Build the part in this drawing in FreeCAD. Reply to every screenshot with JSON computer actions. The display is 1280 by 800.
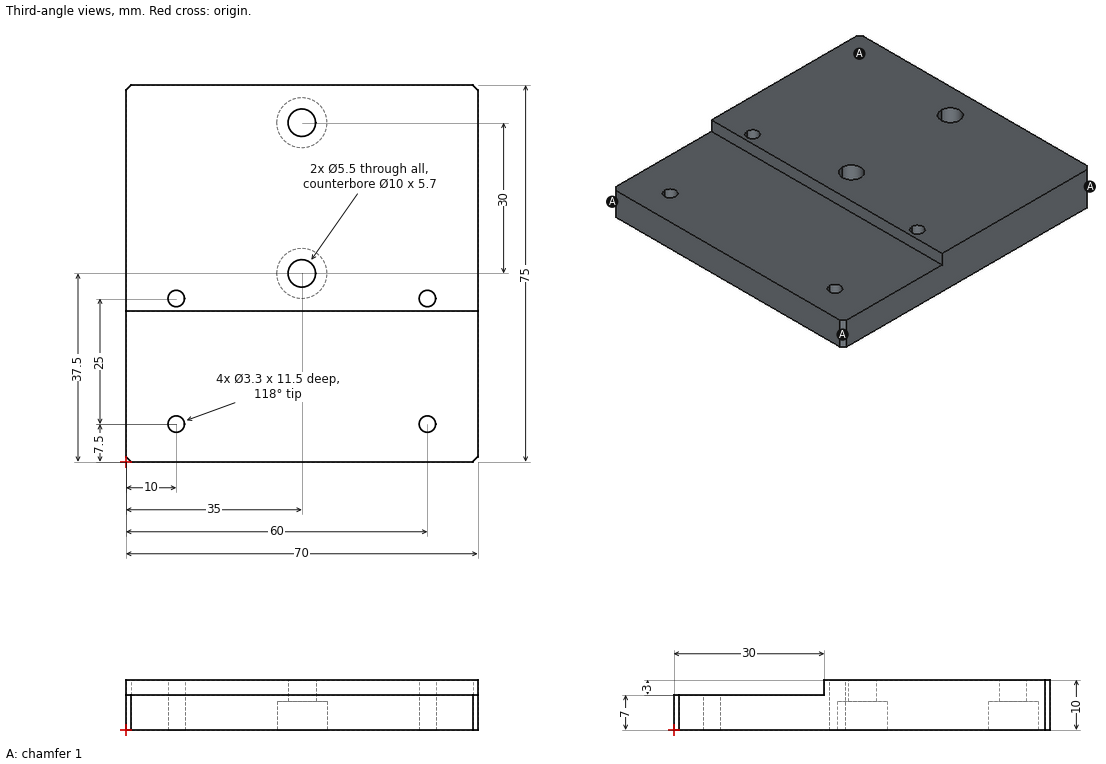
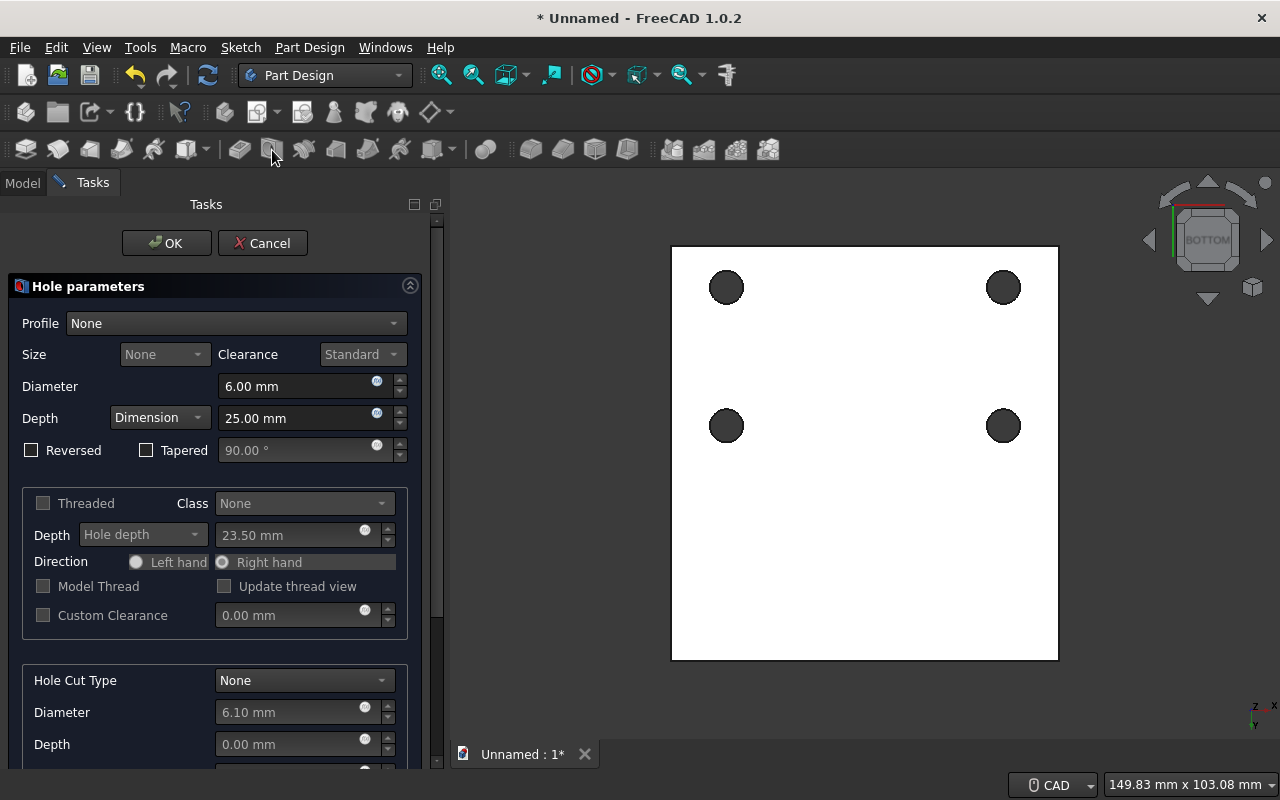
{"action": "triple_click", "coordinate": [305, 386]}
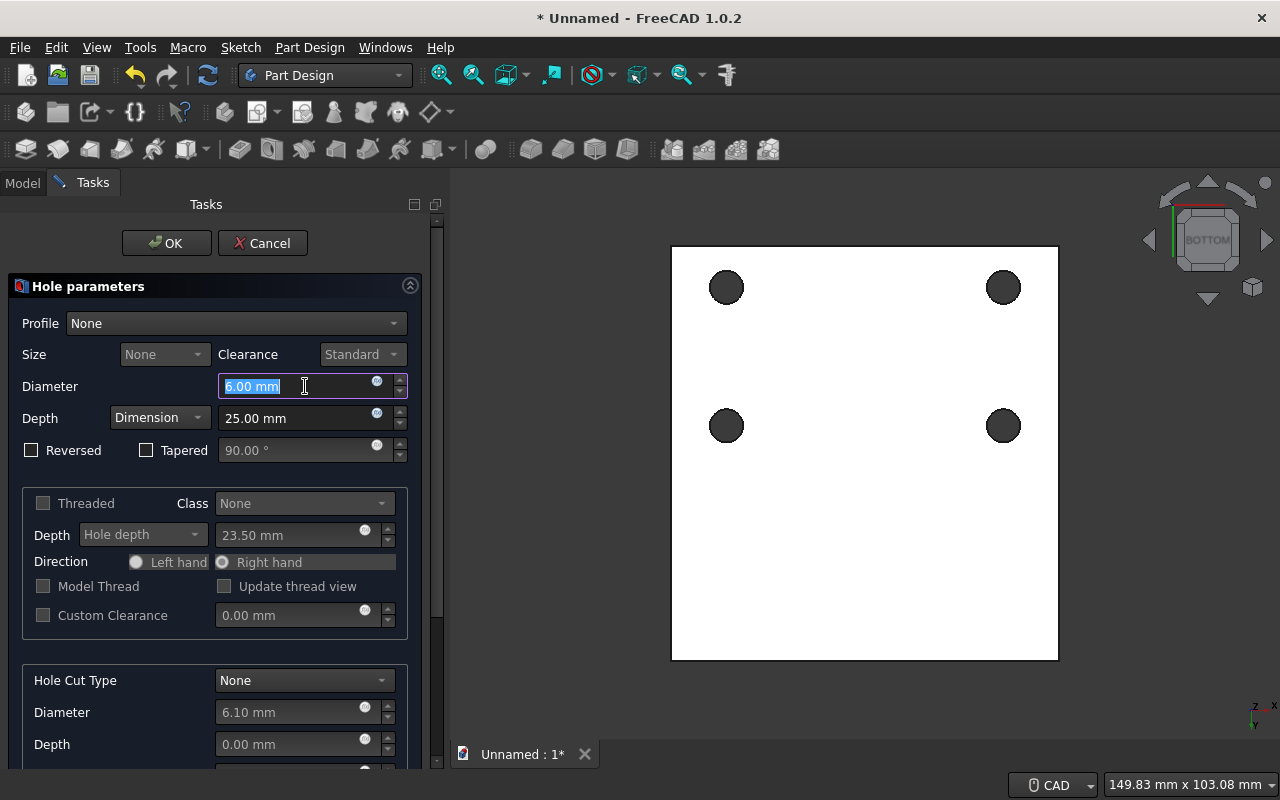
{"action": "type", "text": "3.3"}
{"action": "key", "text": "Tab"}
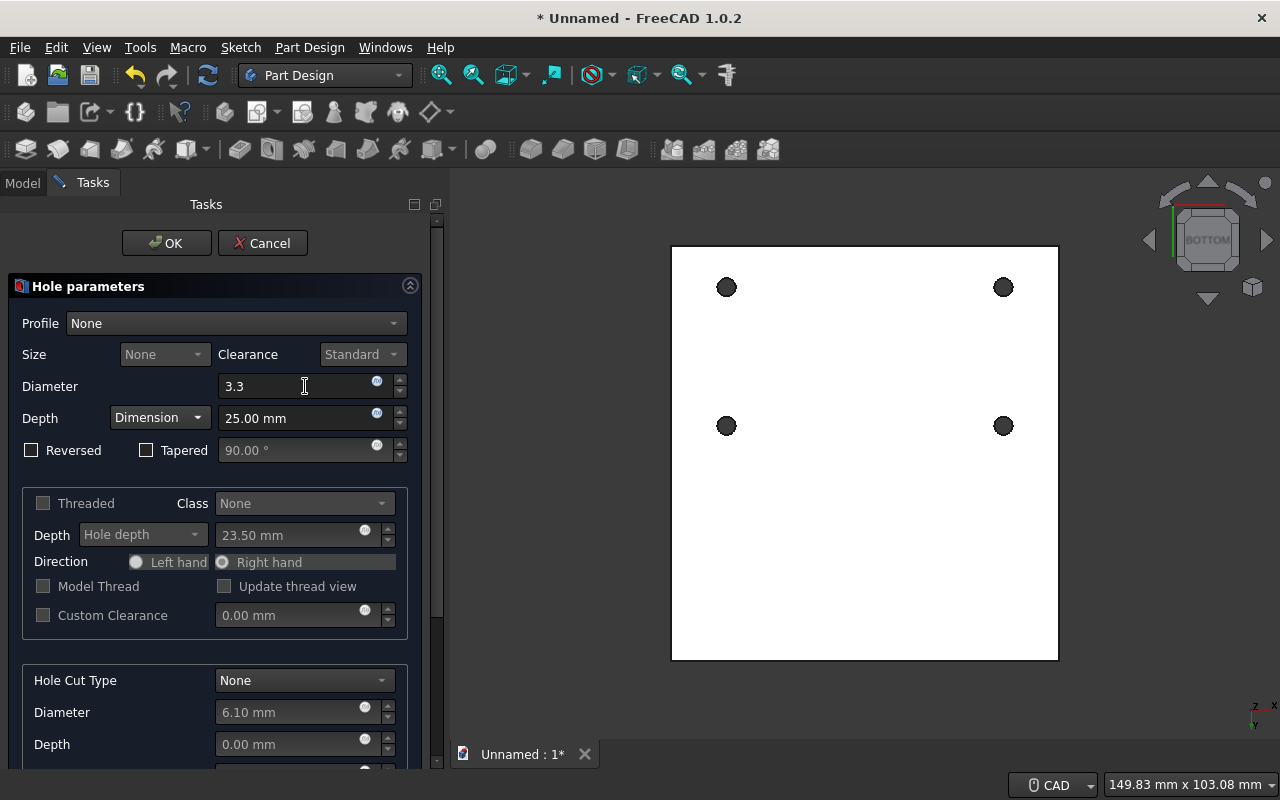
{"action": "triple_click", "coordinate": [305, 418]}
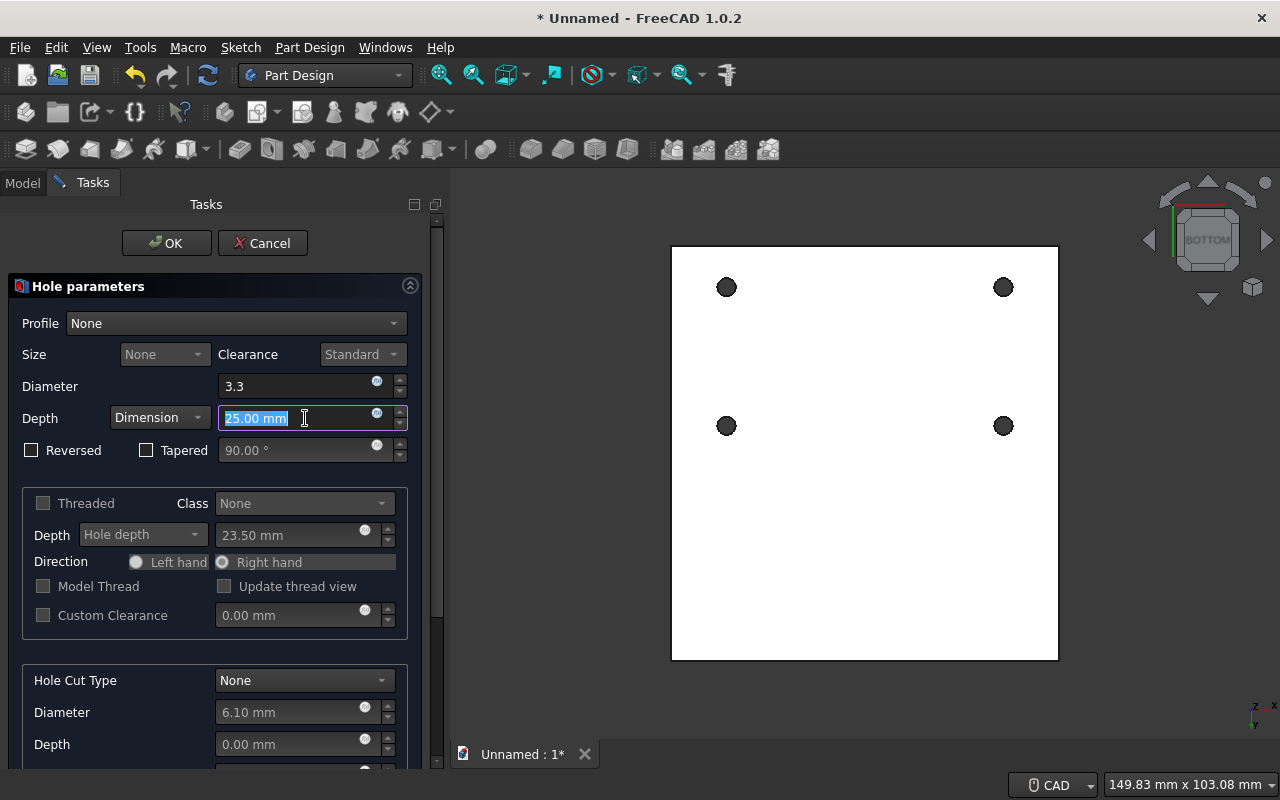
{"action": "type", "text": "11.5"}
{"action": "key", "text": "Tab"}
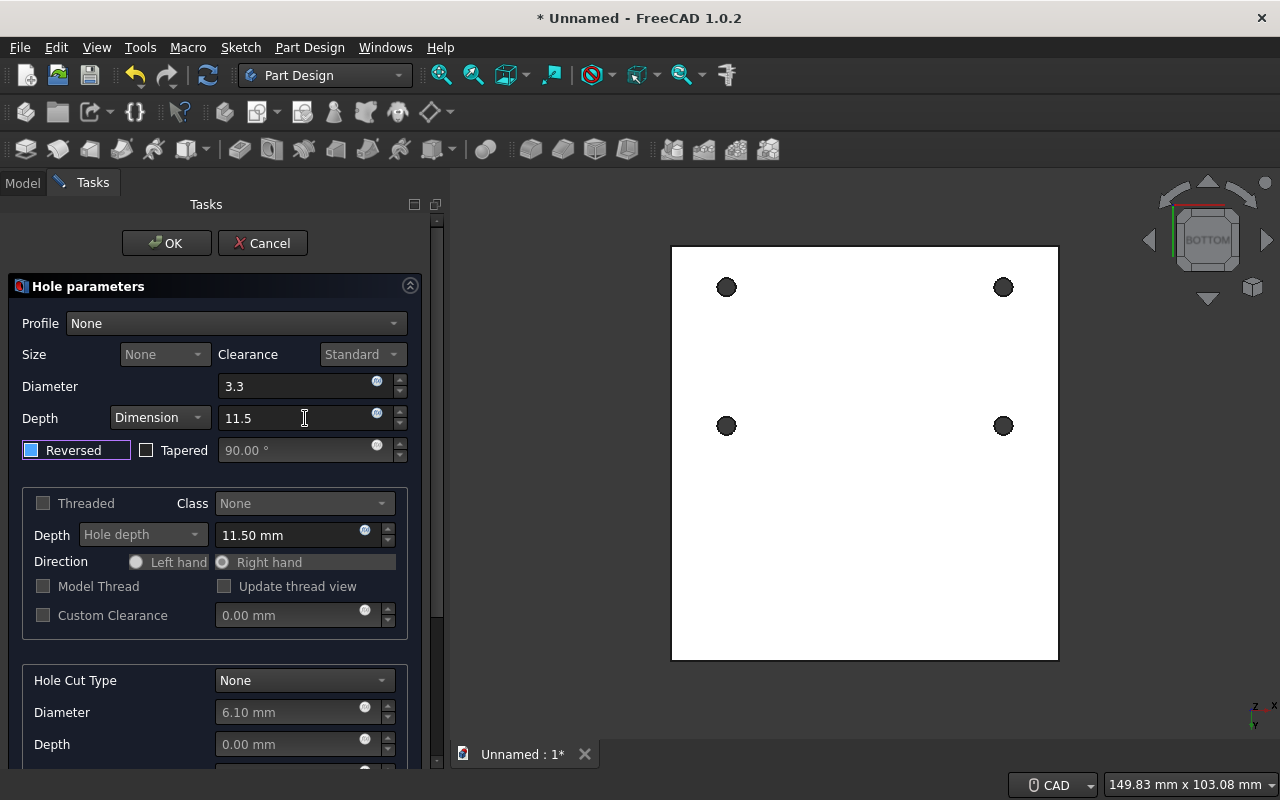
{"action": "left_click", "coordinate": [167, 243]}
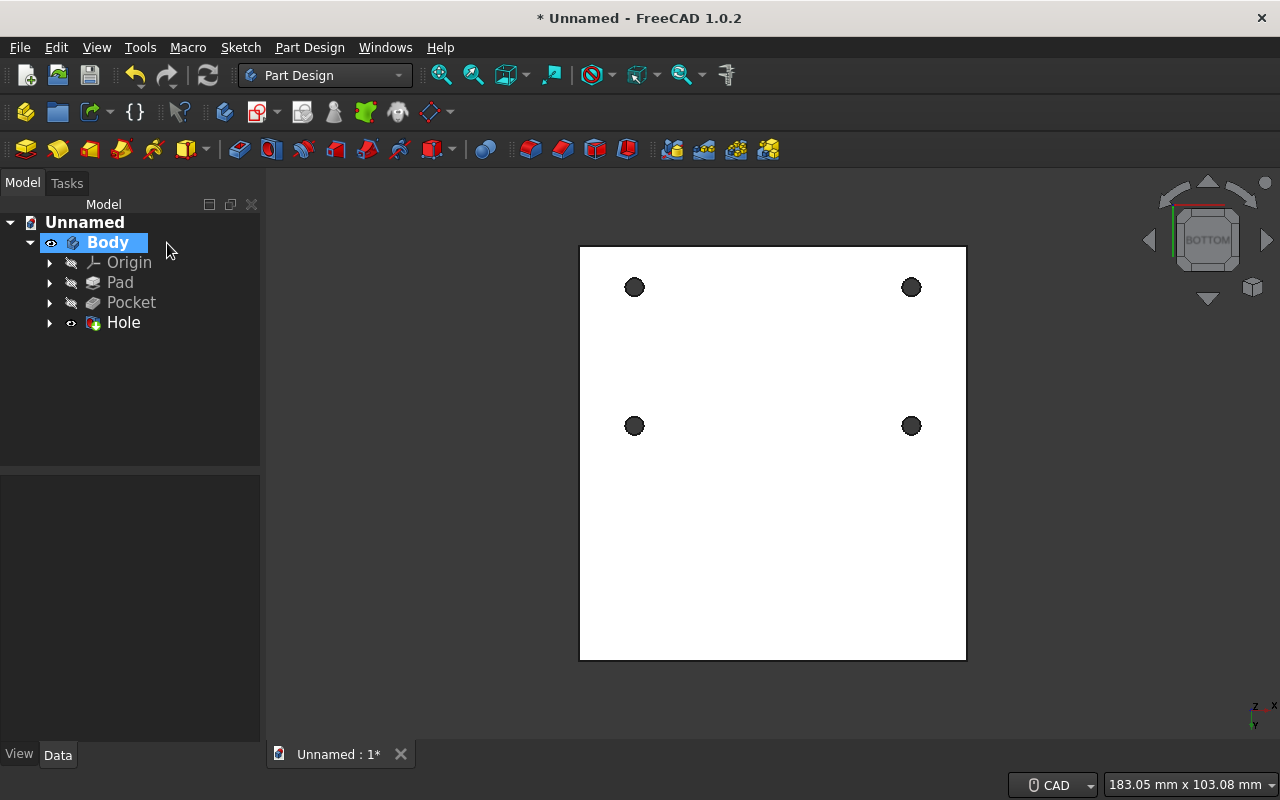
{"action": "left_click", "coordinate": [258, 112]}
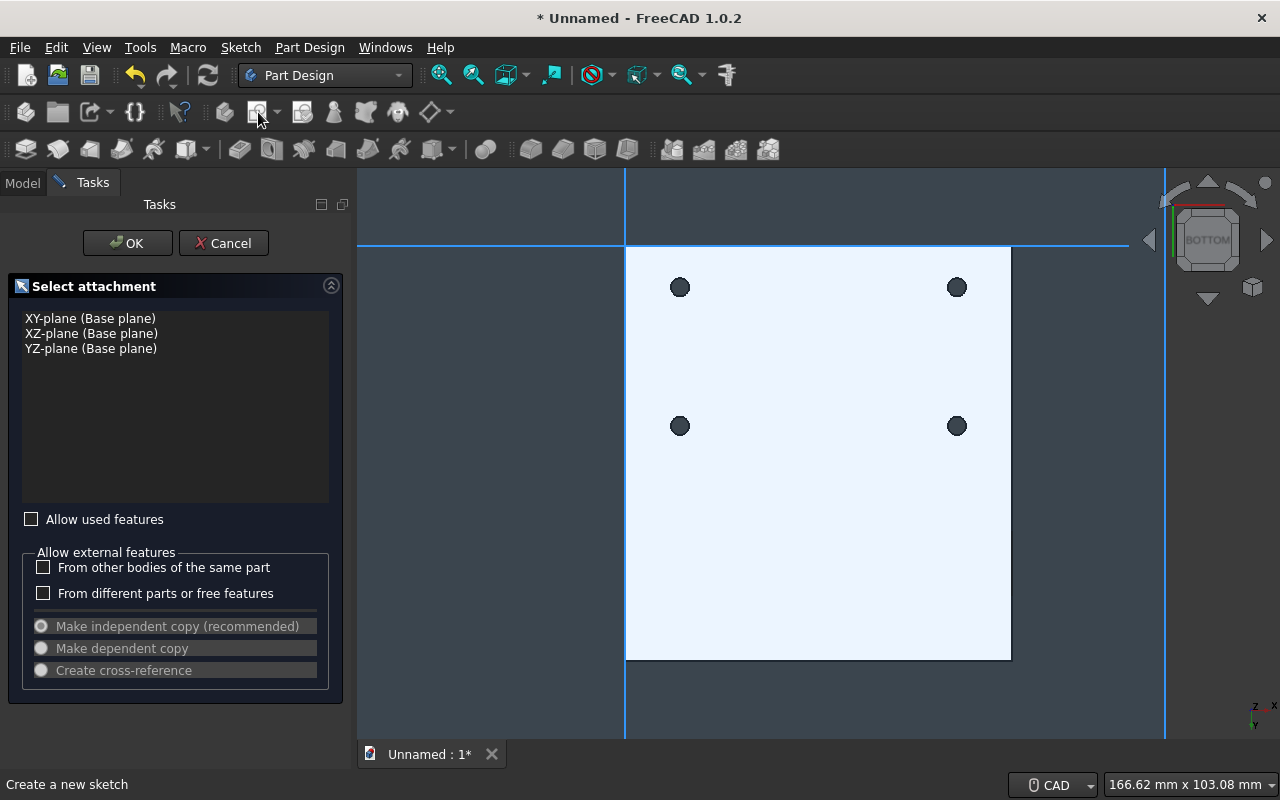
{"action": "left_click", "coordinate": [82, 318]}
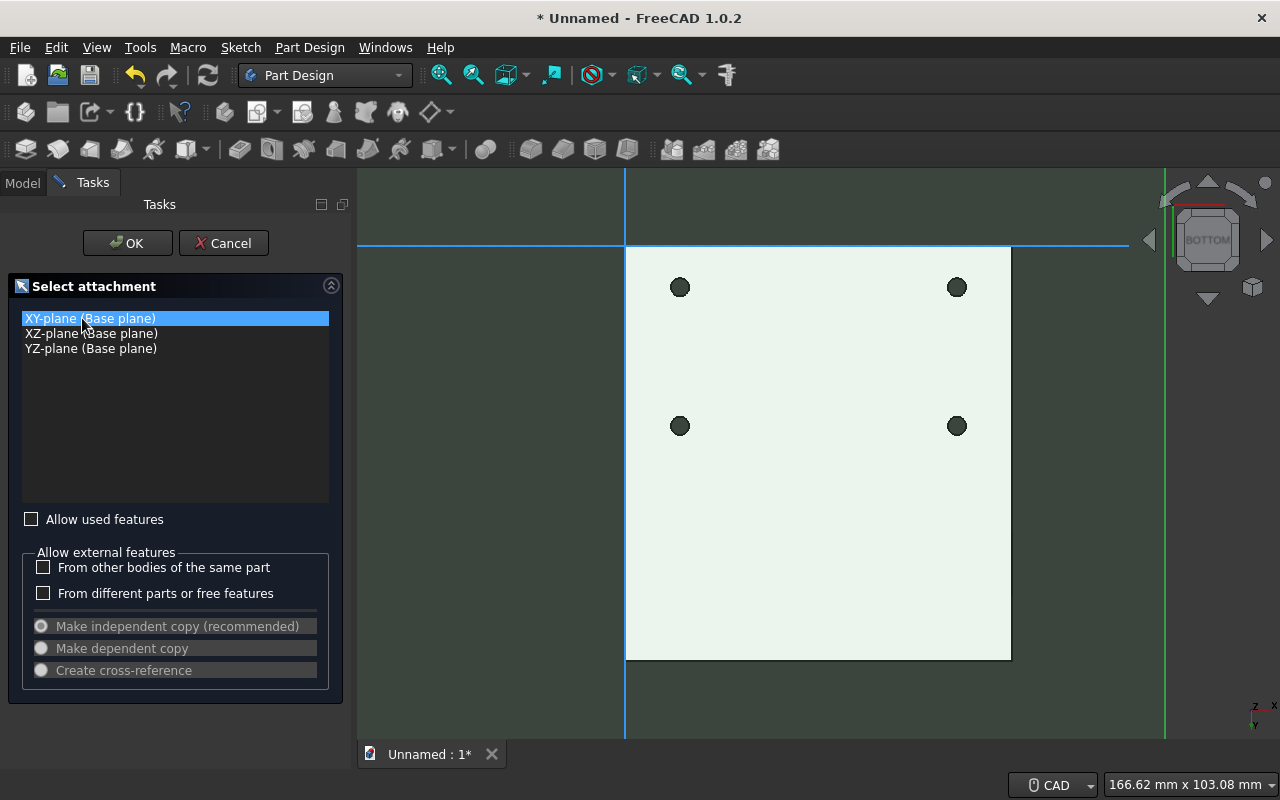
{"action": "left_click", "coordinate": [128, 243]}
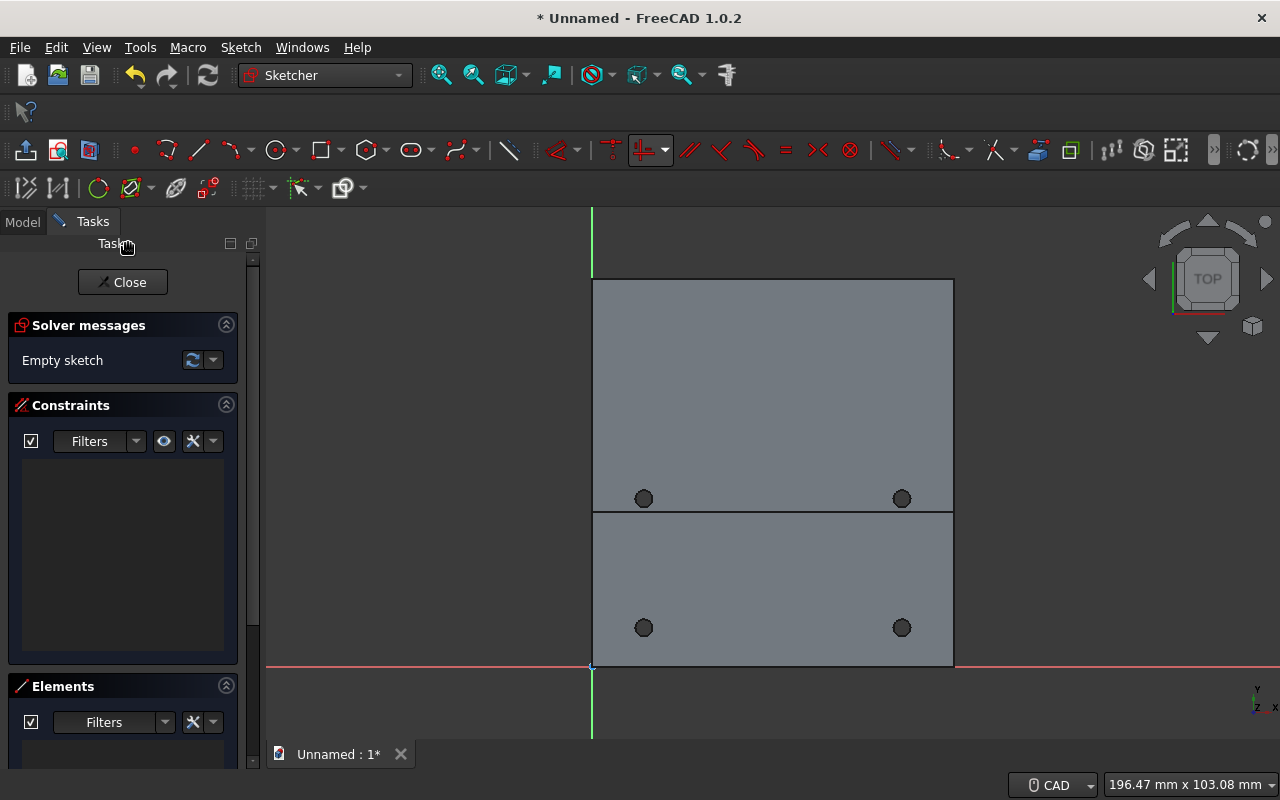
{"action": "key", "text": "q s"}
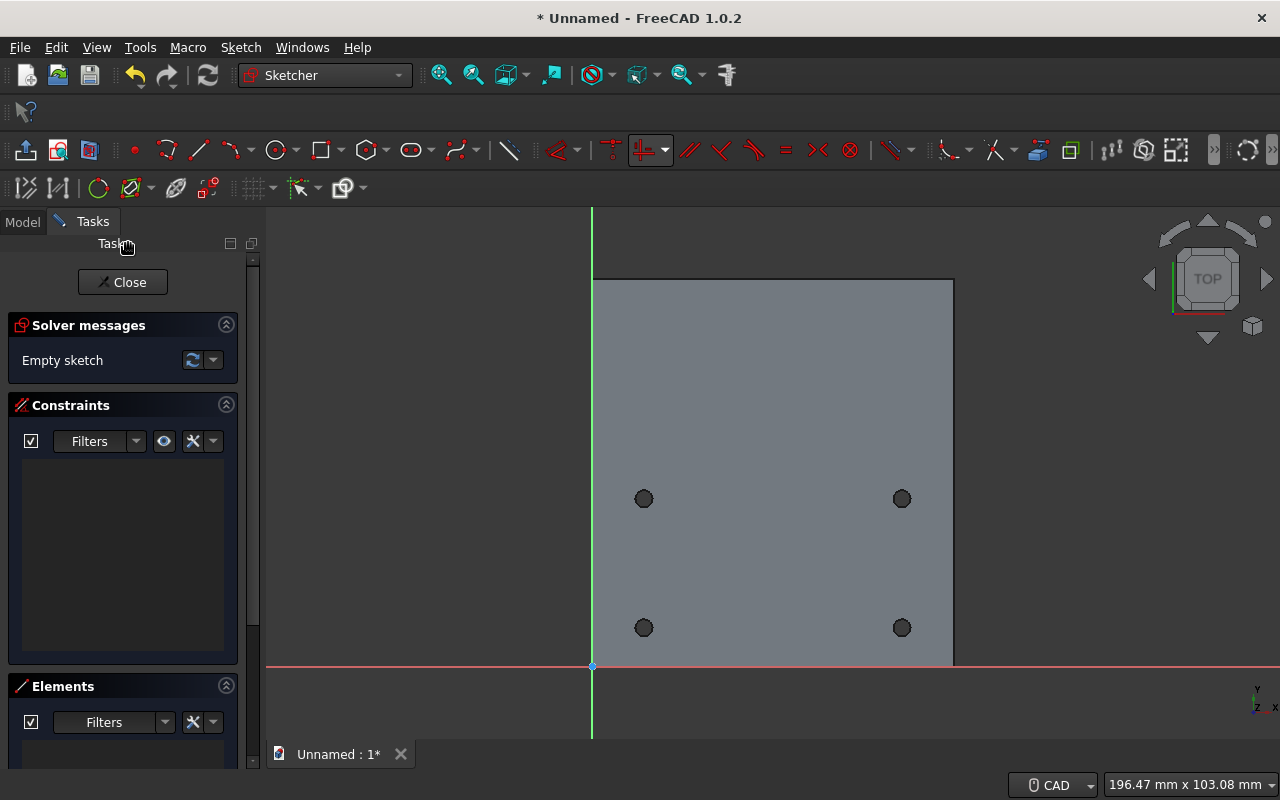
{"action": "left_click", "coordinate": [276, 150]}